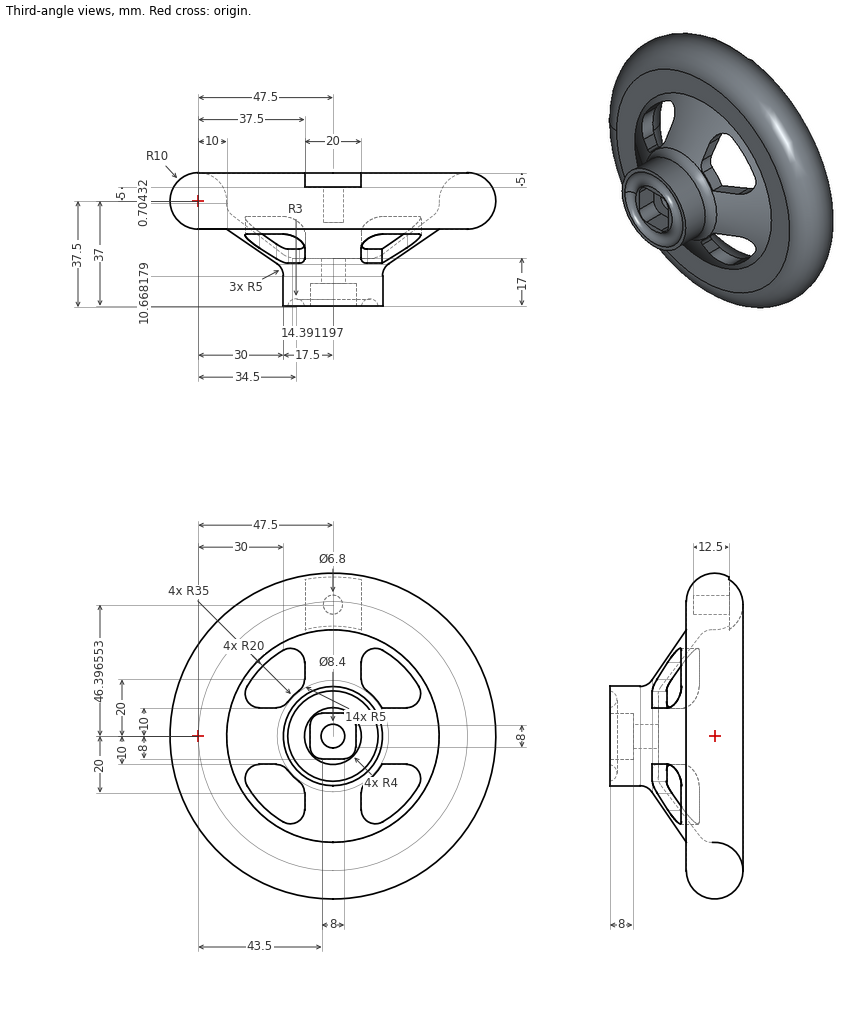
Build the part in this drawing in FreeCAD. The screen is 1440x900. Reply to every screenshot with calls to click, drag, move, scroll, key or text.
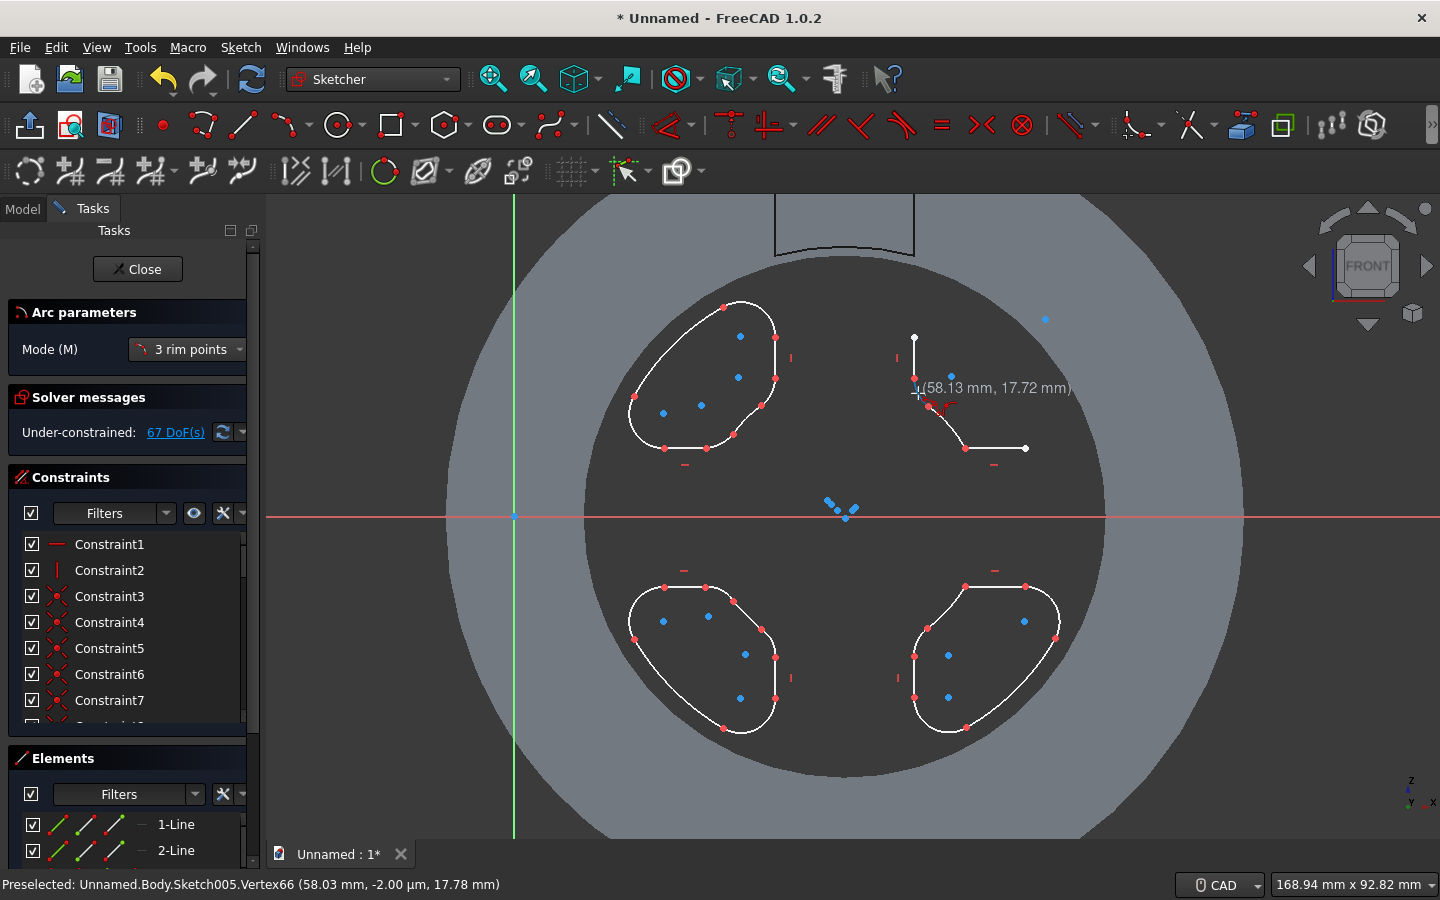
click(914, 337)
click(966, 306)
click(931, 306)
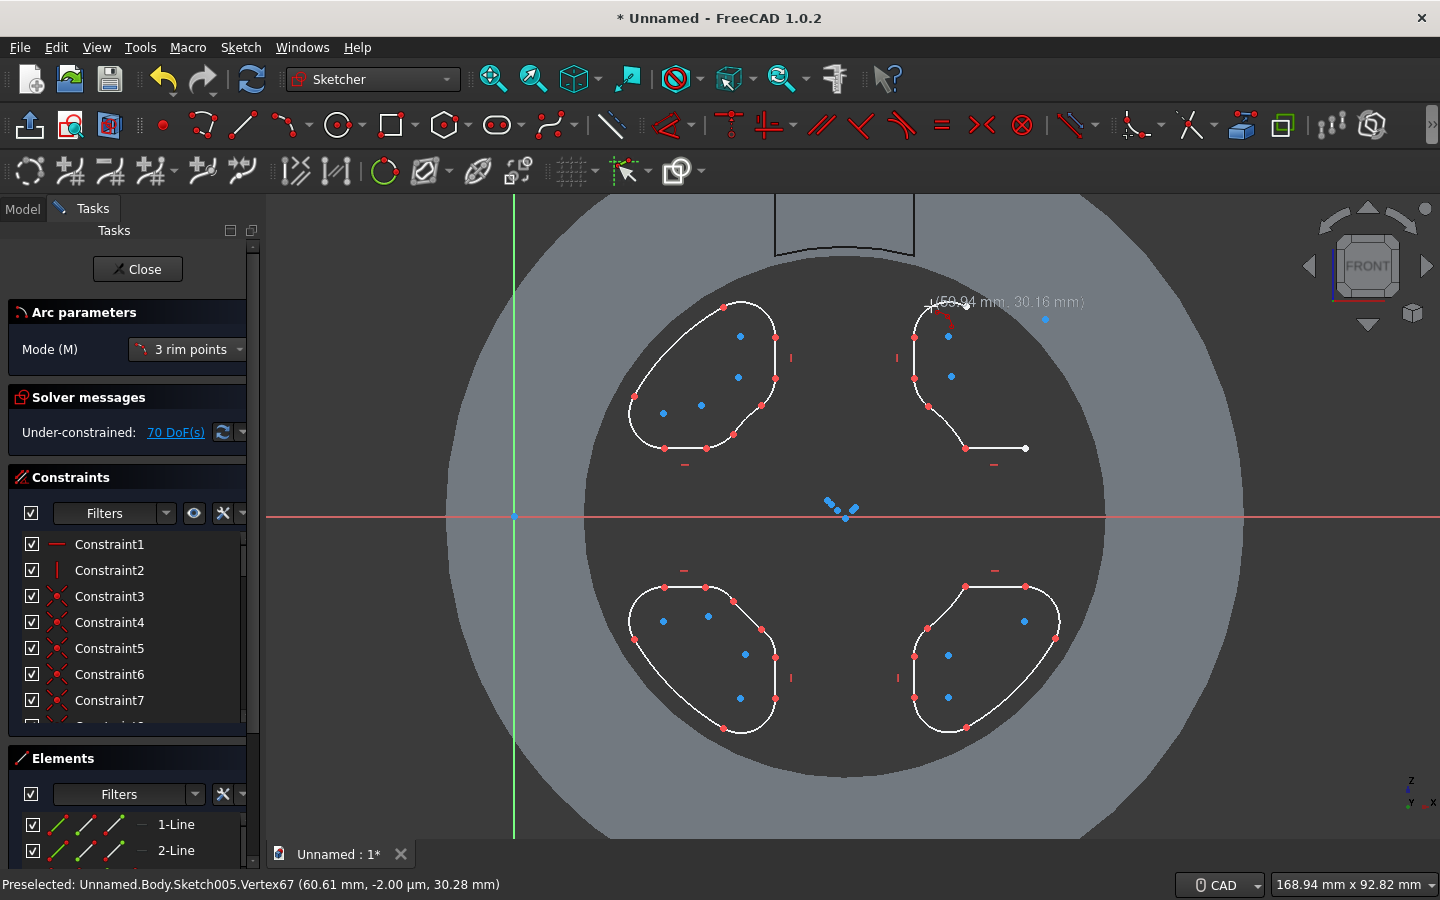
click(966, 307)
click(1055, 395)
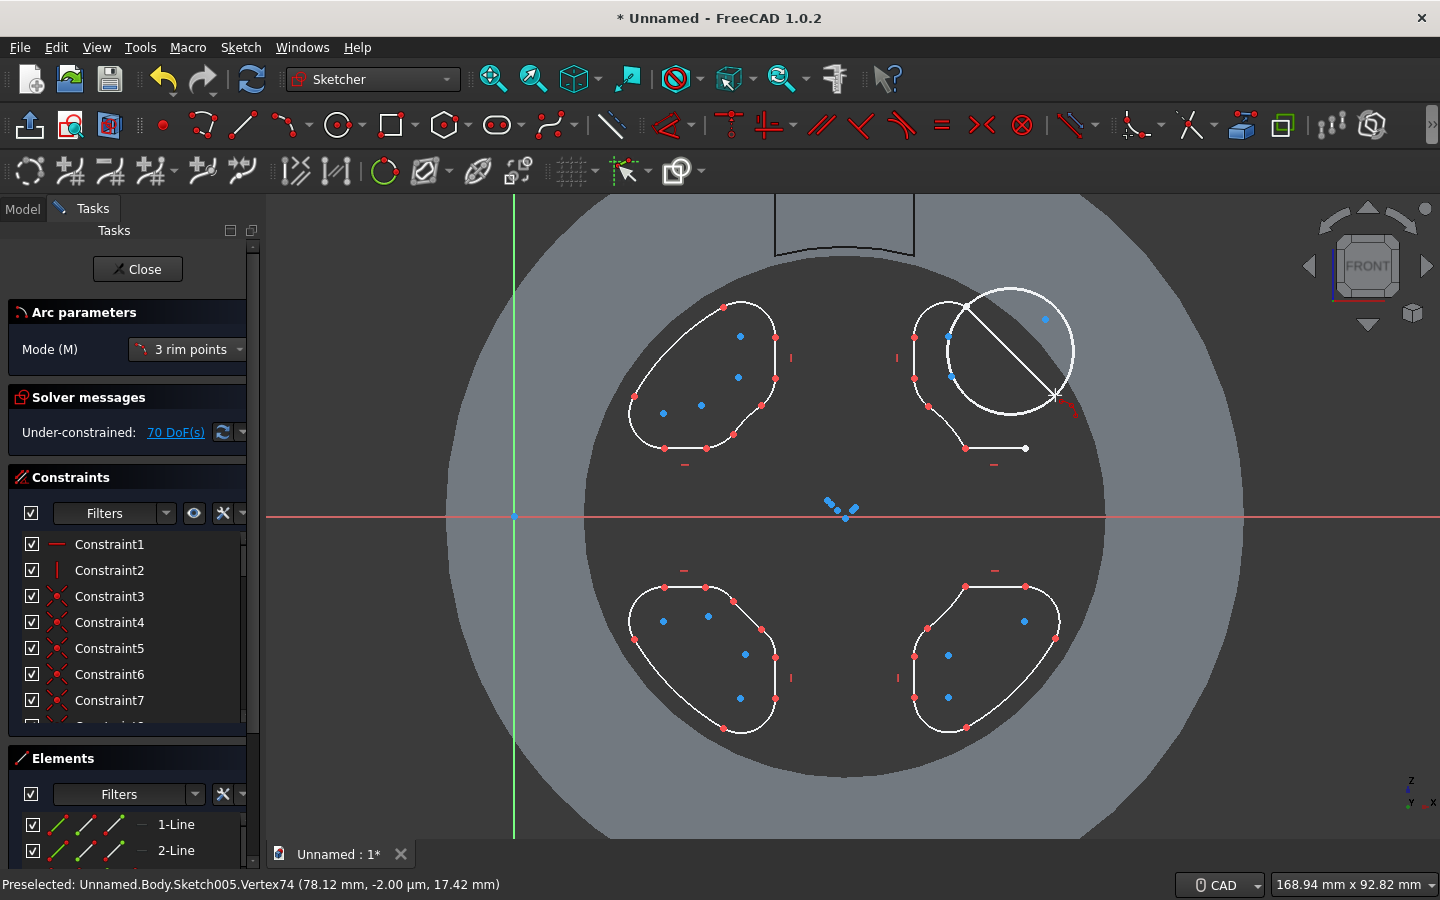
scroll(1017, 345, up, 4)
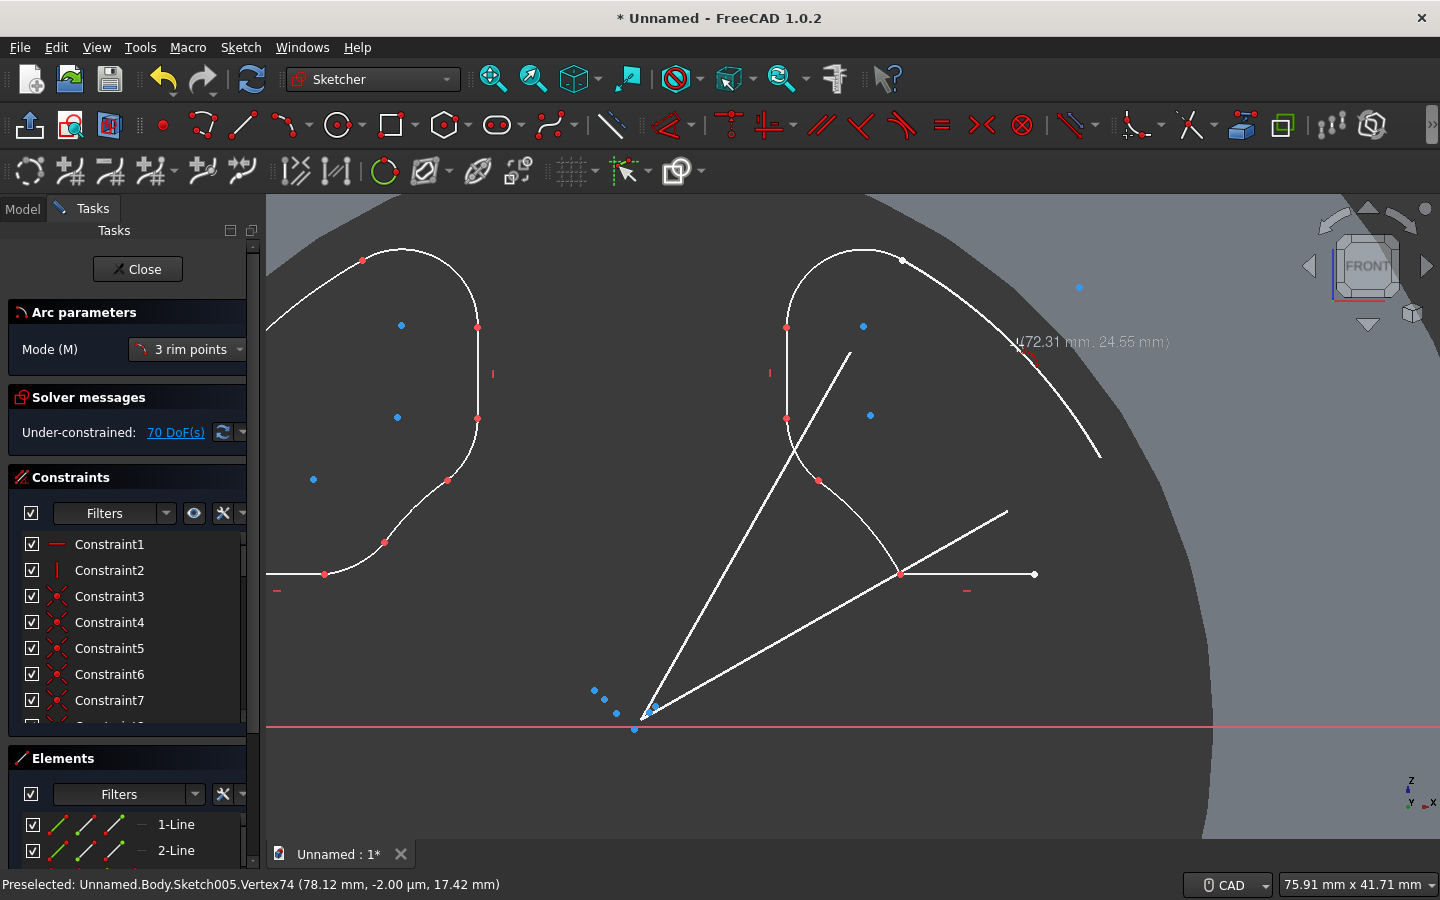
click(1015, 344)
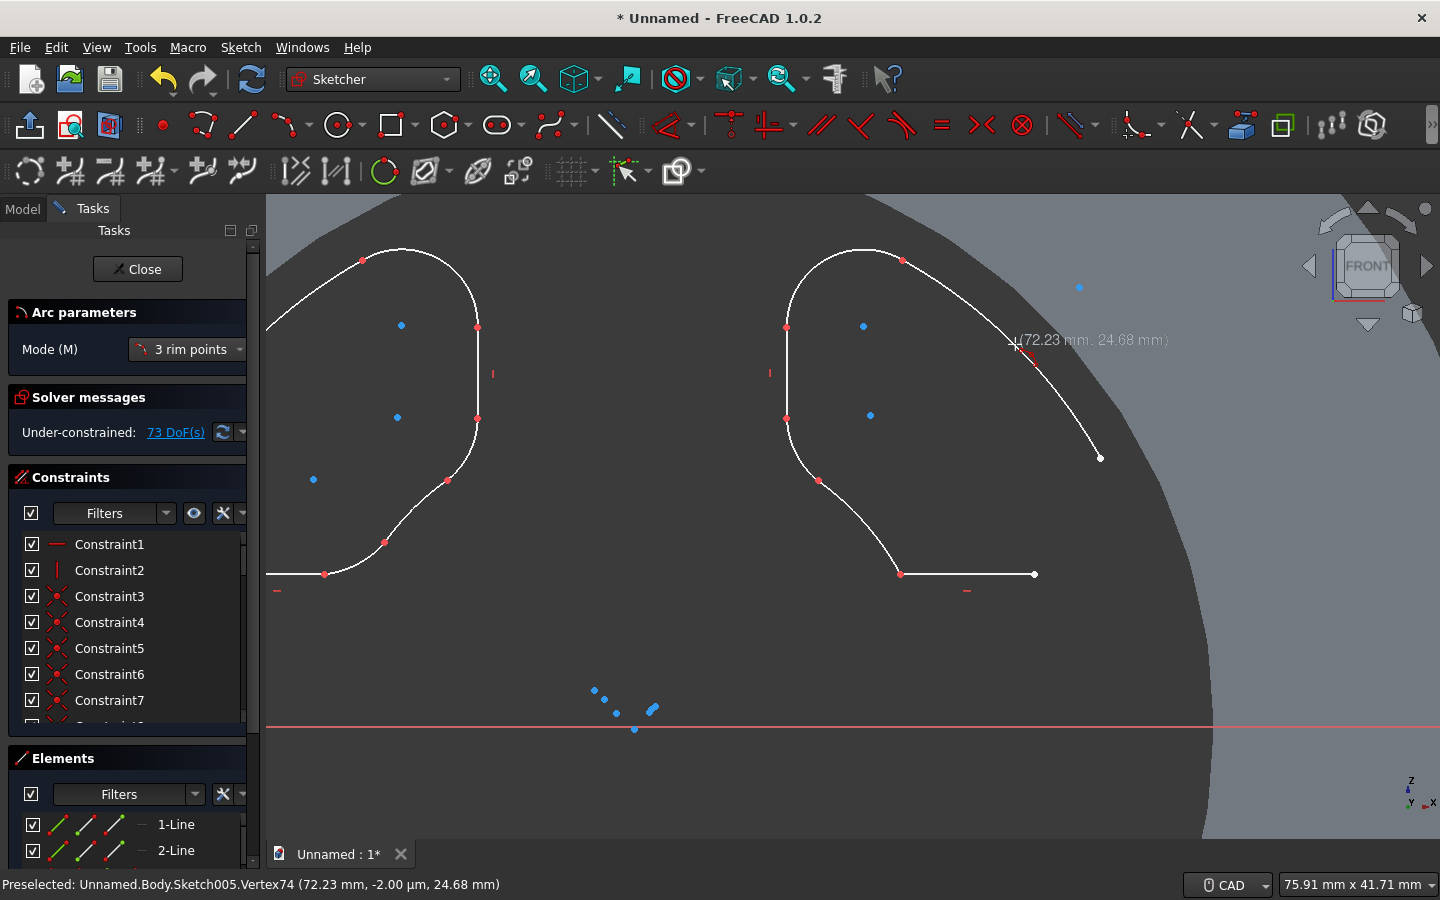
click(1101, 458)
click(1034, 574)
click(1101, 533)
key(Escape)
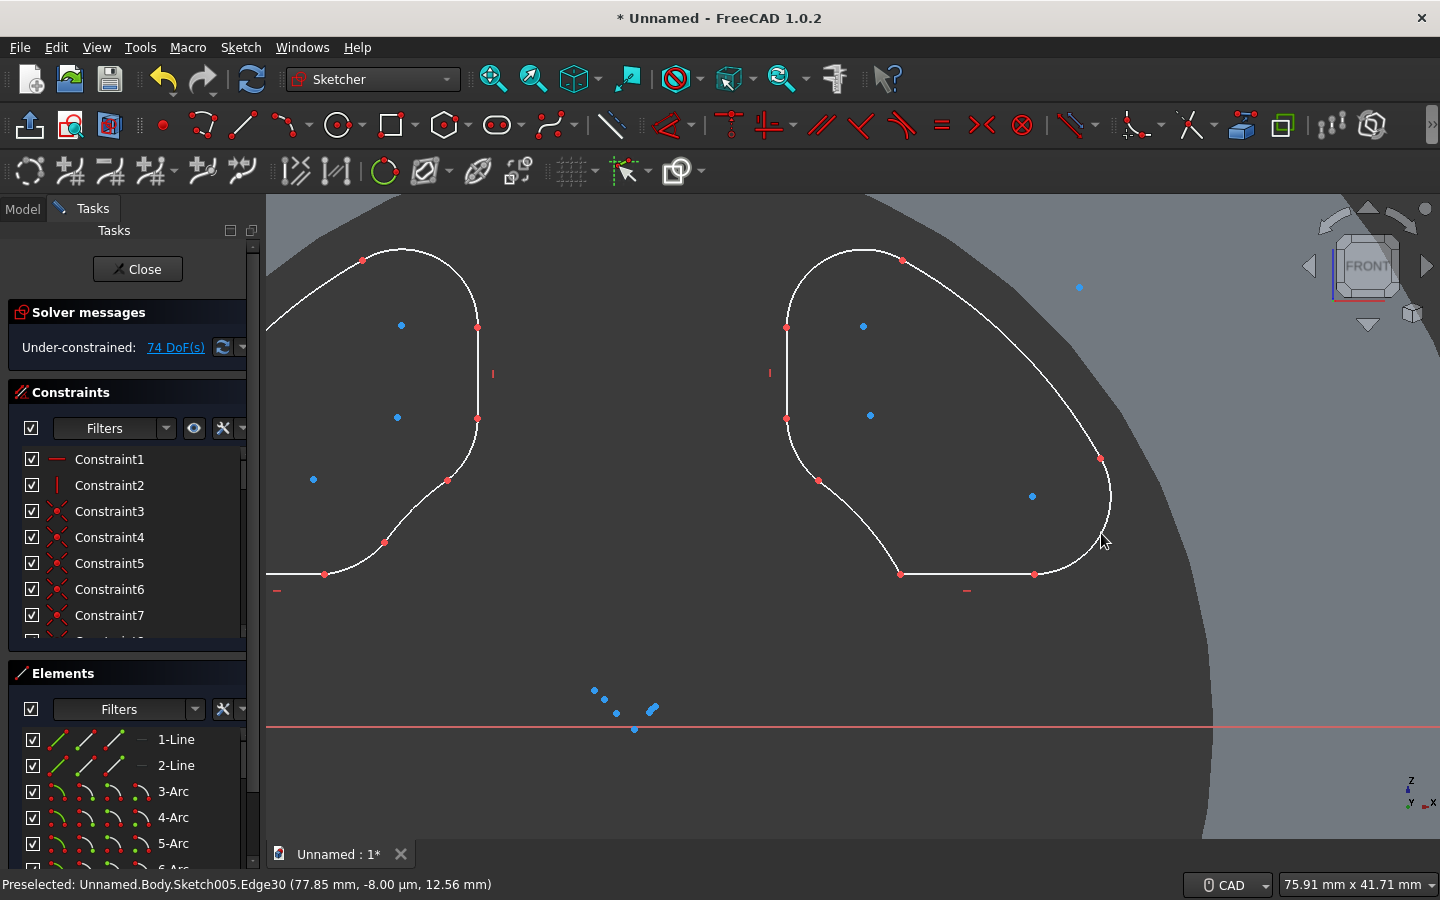
click(296, 574)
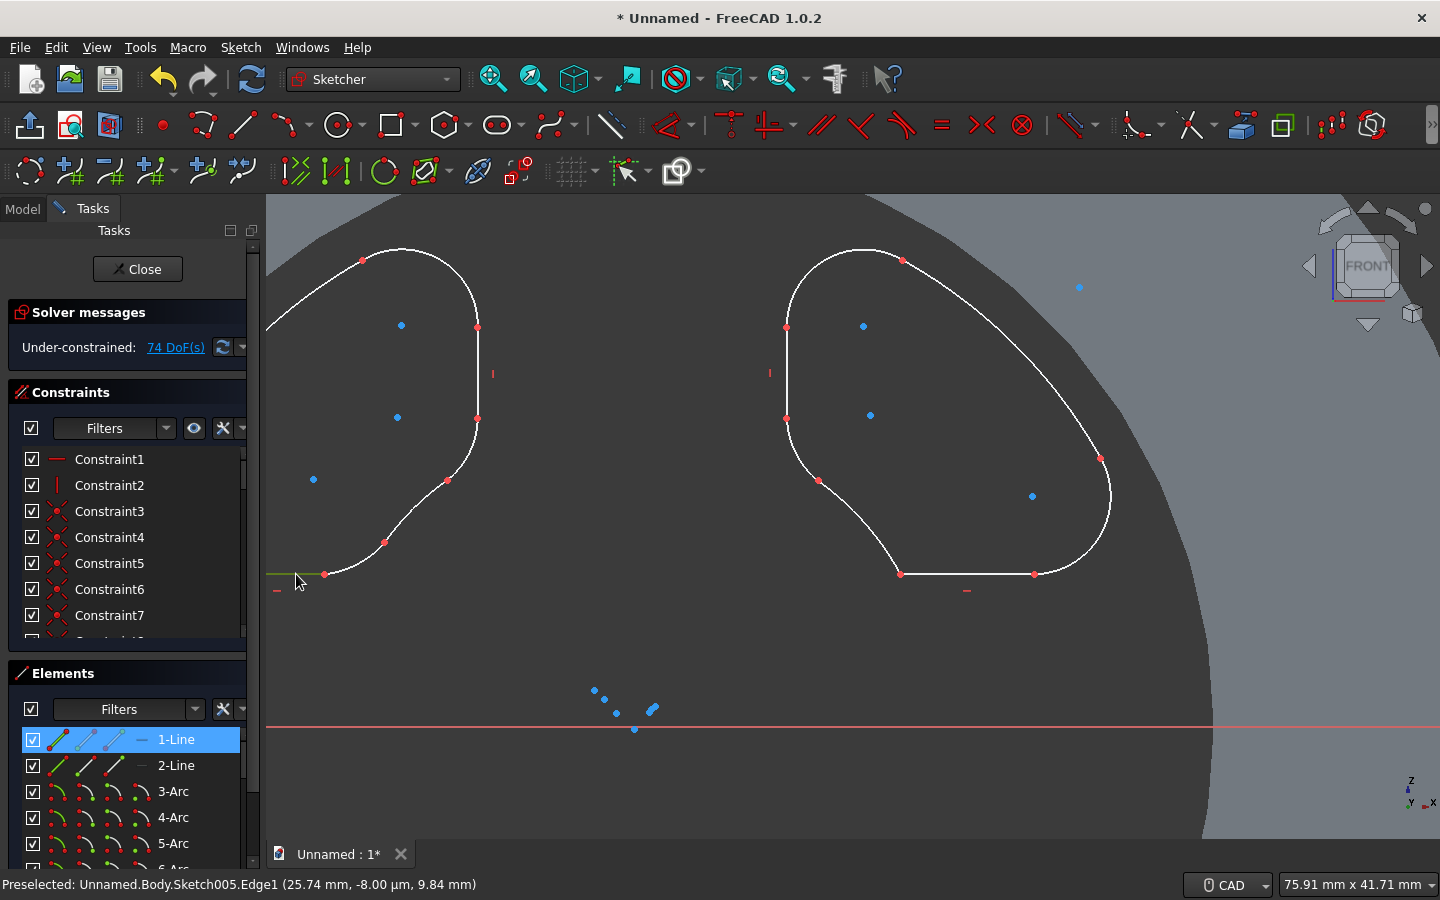
scroll(1017, 345, down, 4)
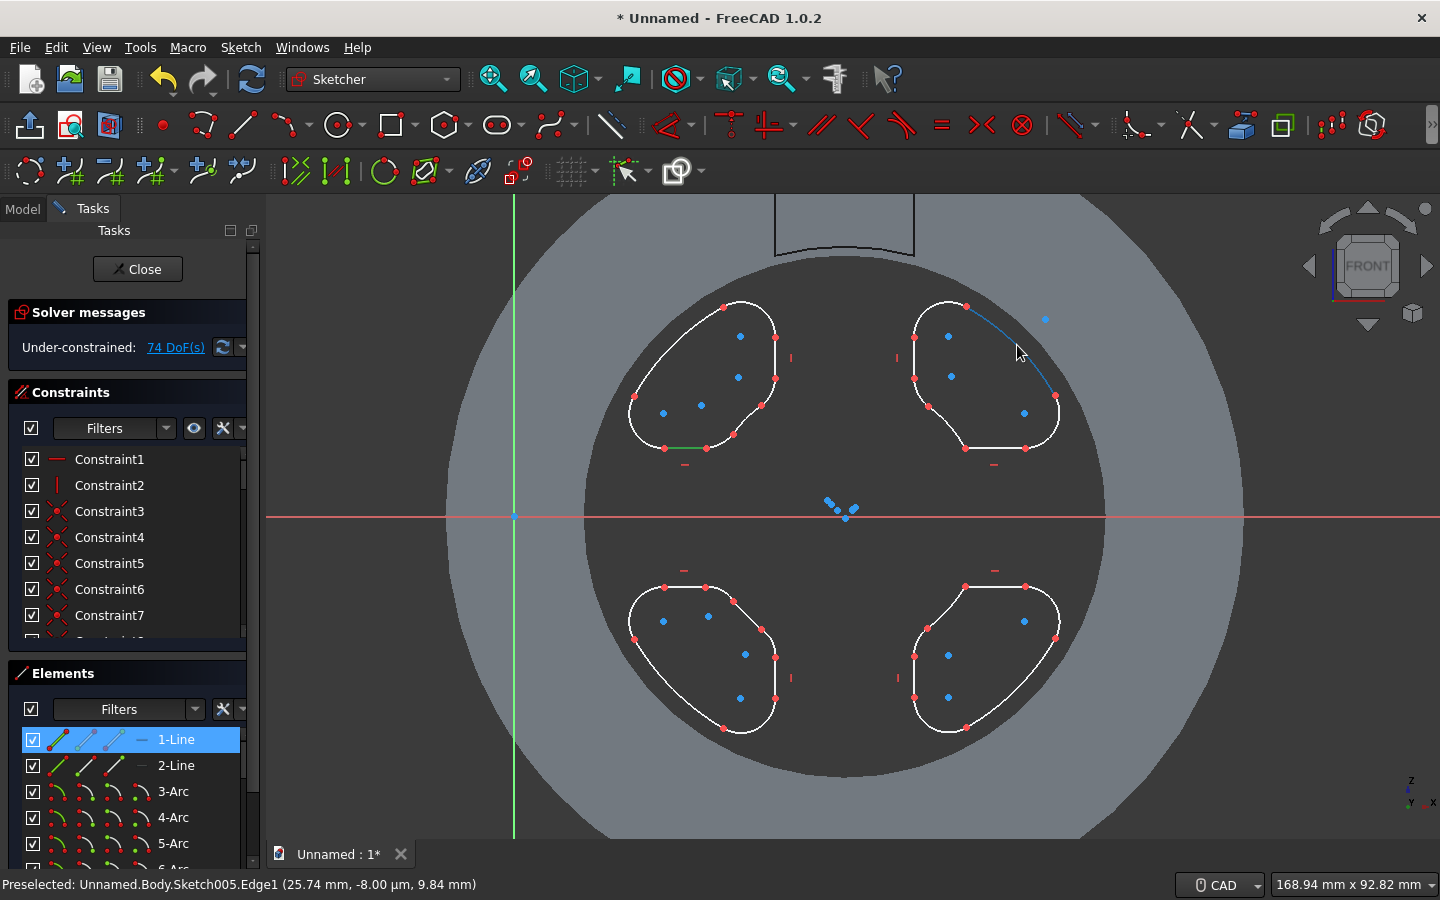
click(629, 417)